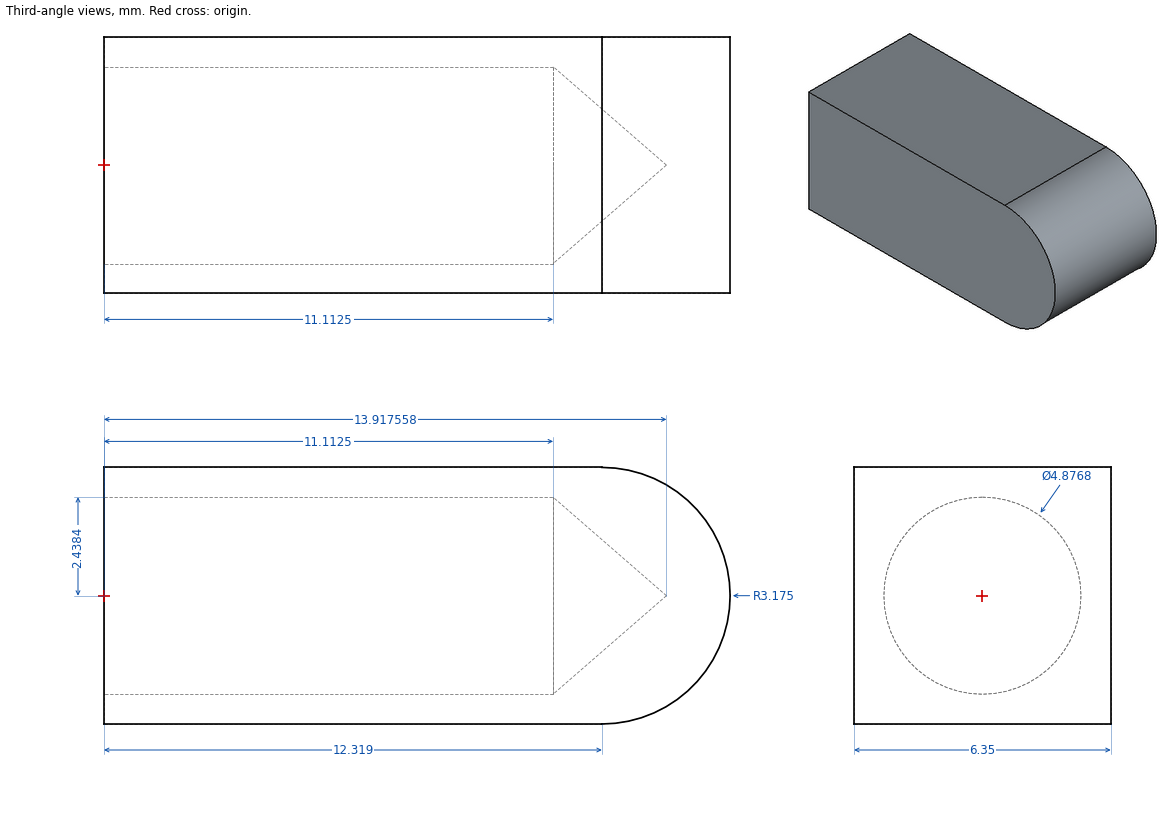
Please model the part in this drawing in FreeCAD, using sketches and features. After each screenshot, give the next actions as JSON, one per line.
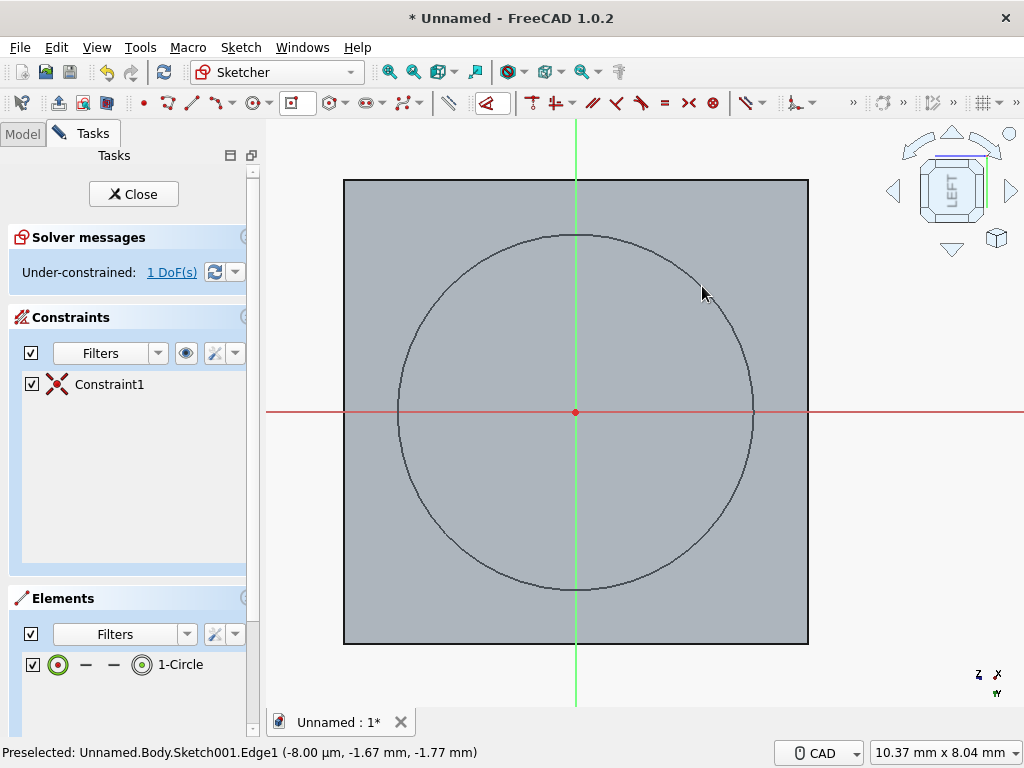
{"action": "key", "text": "d"}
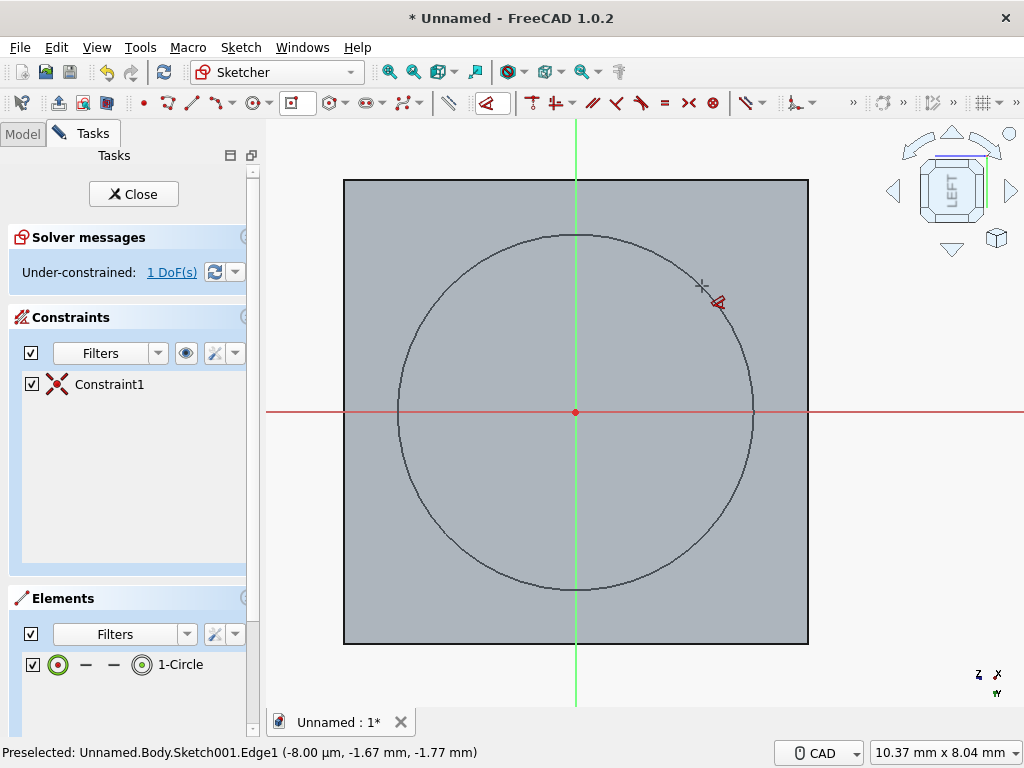
{"action": "left_click", "coordinate": [701, 286]}
{"action": "left_click", "coordinate": [724, 263]}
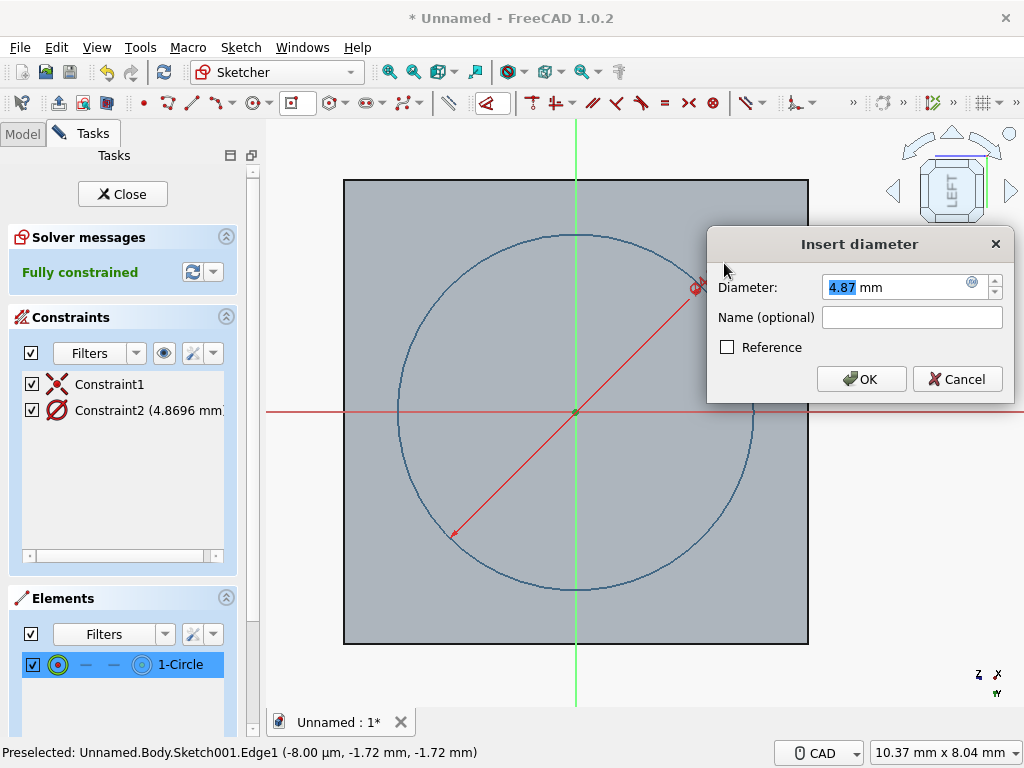
{"action": "type", "text": "4.8768"}
{"action": "key", "text": "Return"}
{"action": "key", "text": "Escape"}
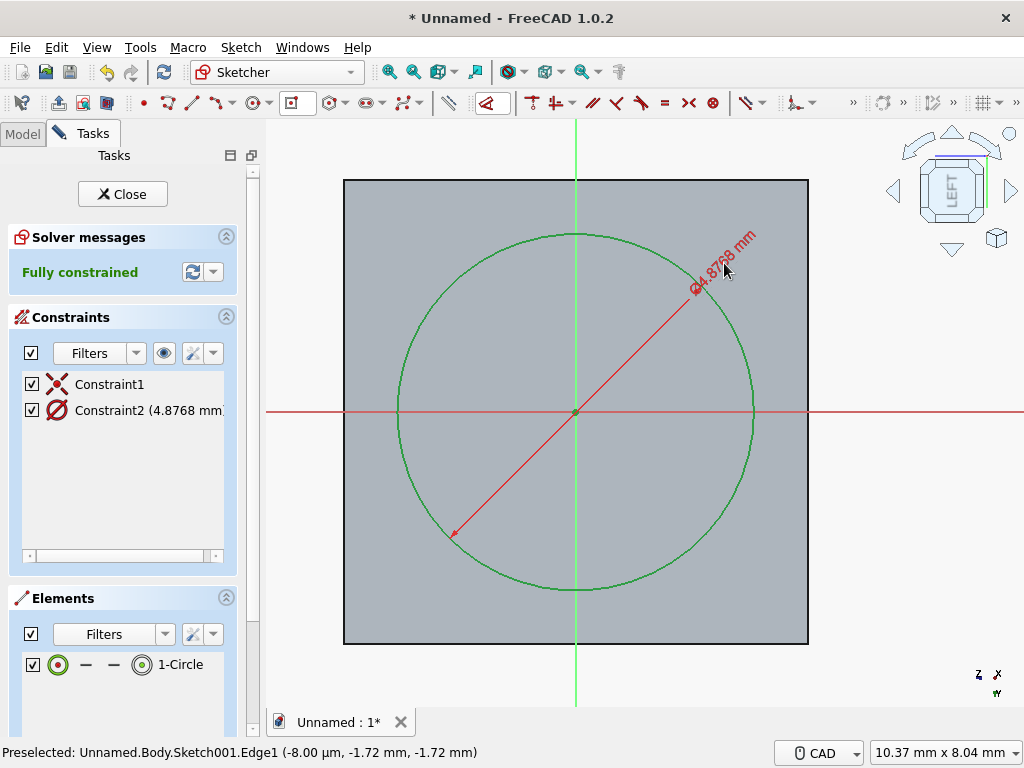
{"action": "left_click", "coordinate": [123, 194]}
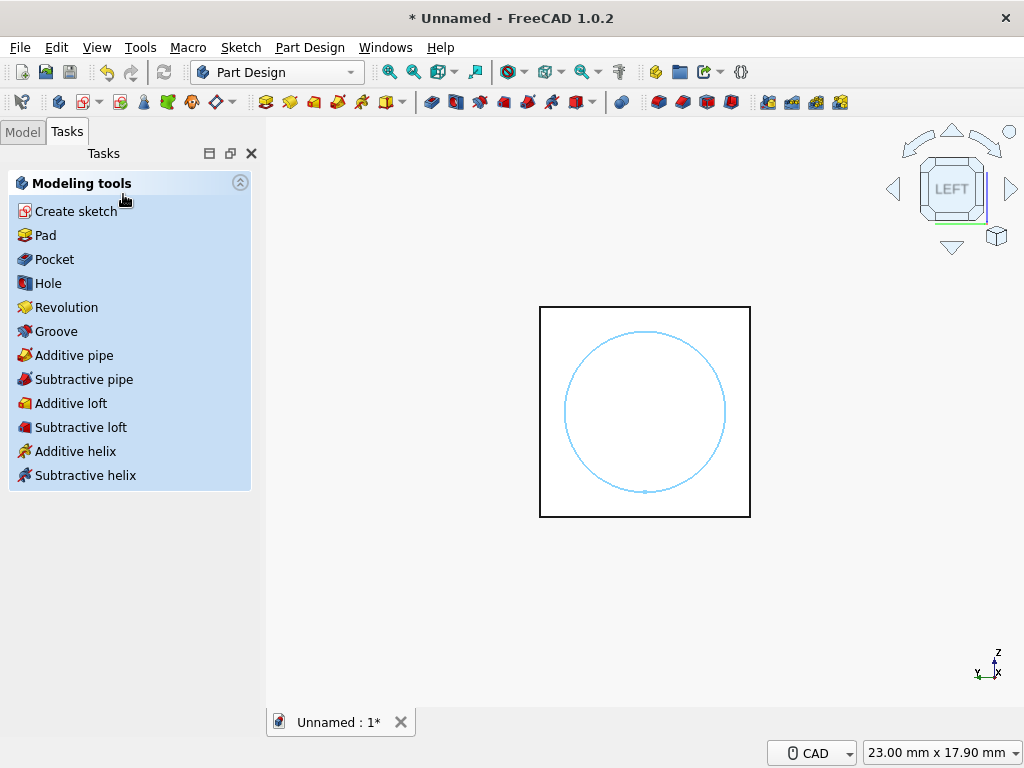
{"action": "left_click", "coordinate": [432, 102]}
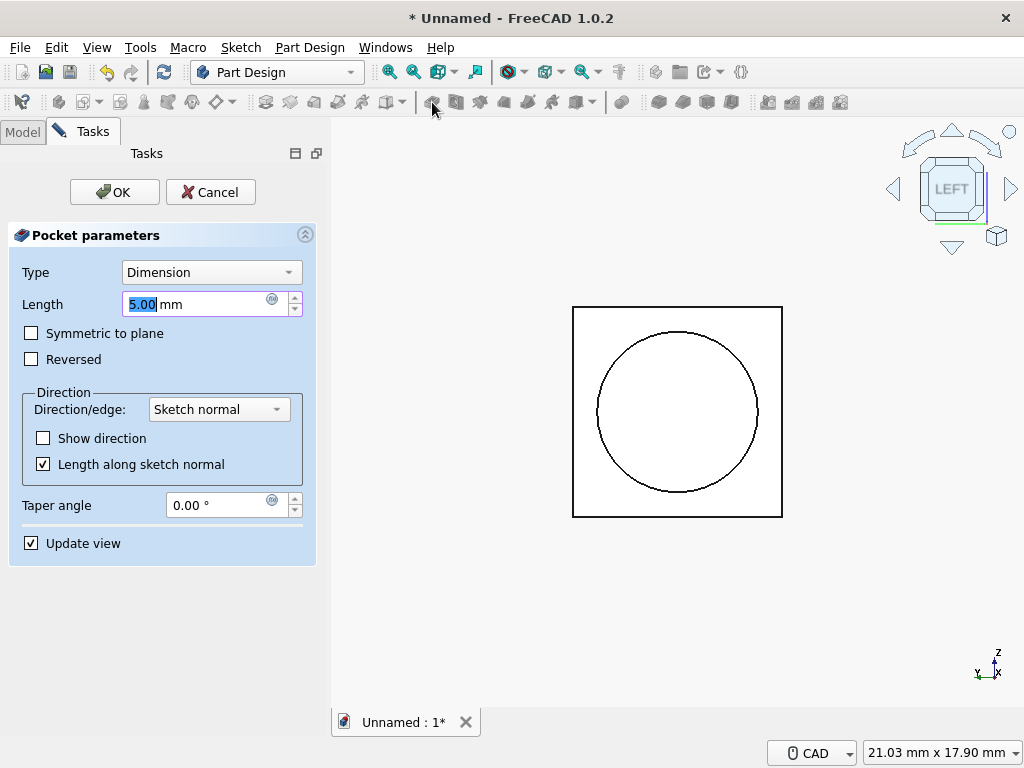
{"action": "type", "text": "11.1125"}
{"action": "key", "text": "Tab"}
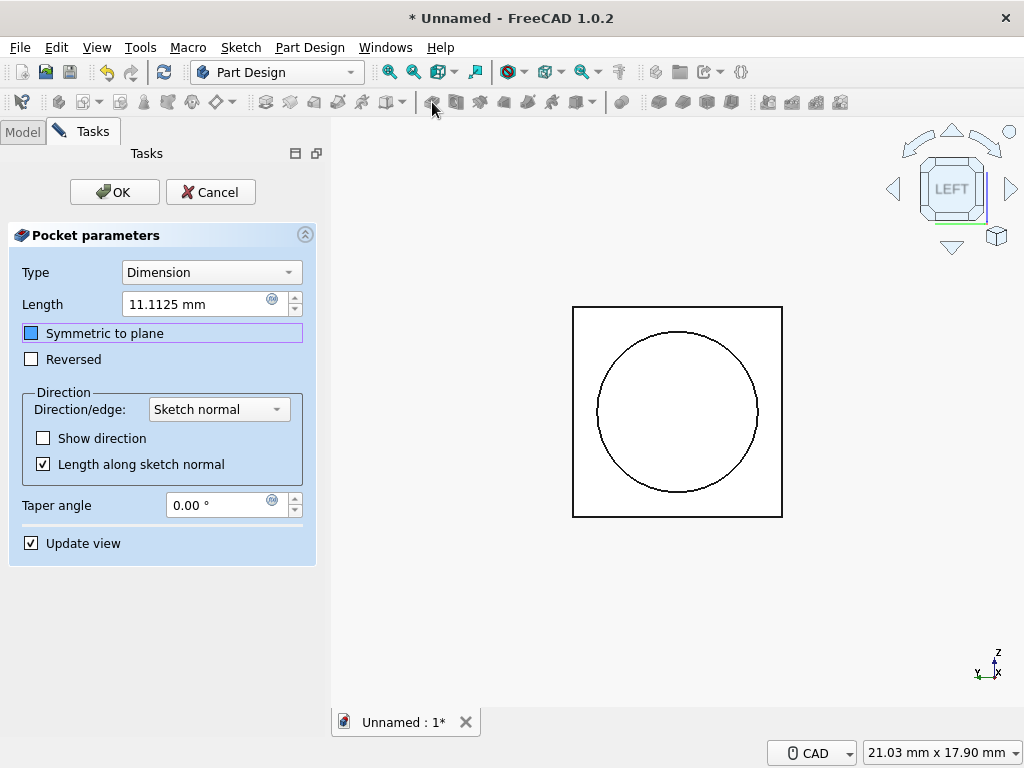
{"action": "left_click", "coordinate": [115, 192]}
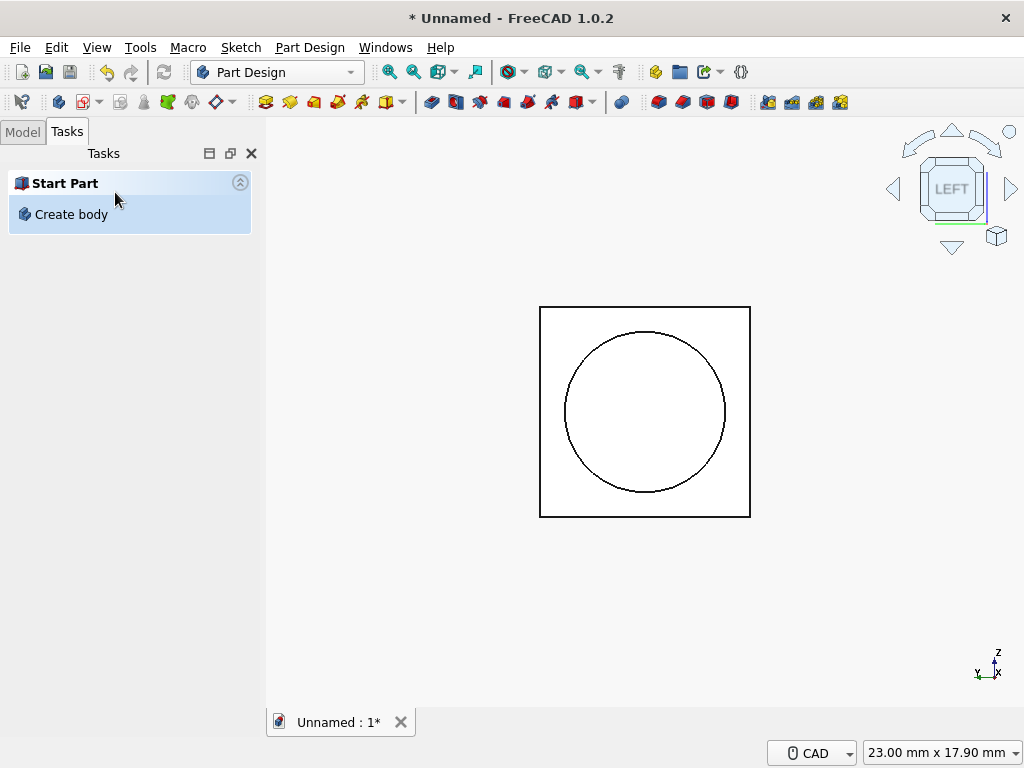
{"action": "key", "text": "v f"}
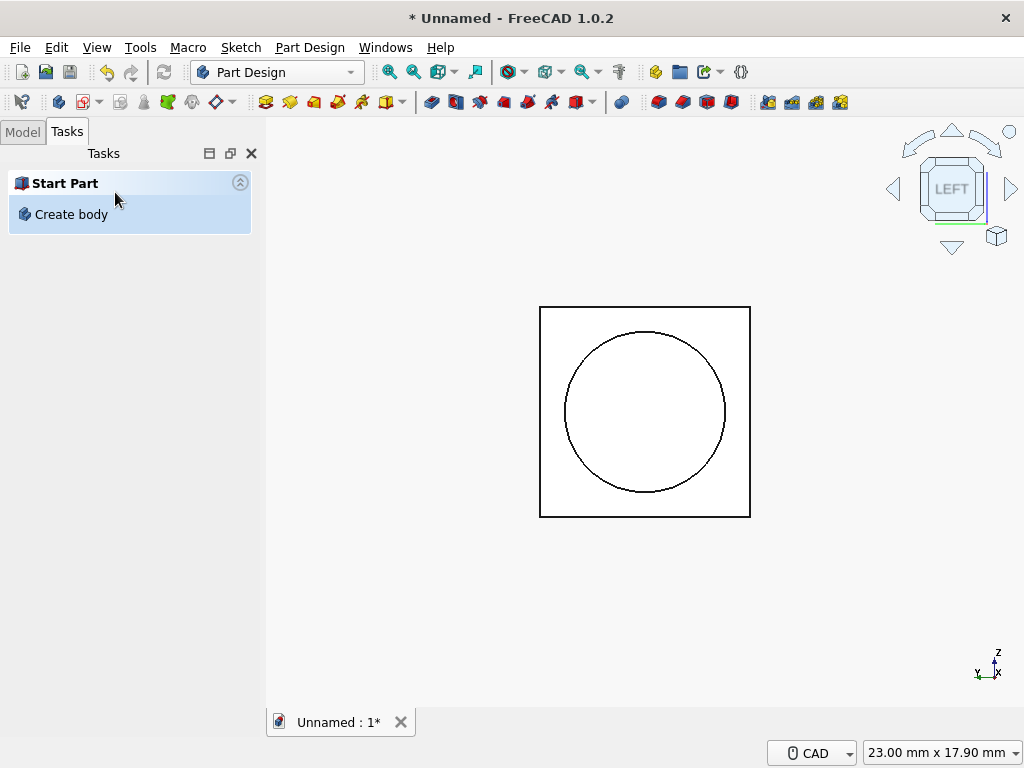
{"action": "left_click", "coordinate": [84, 102]}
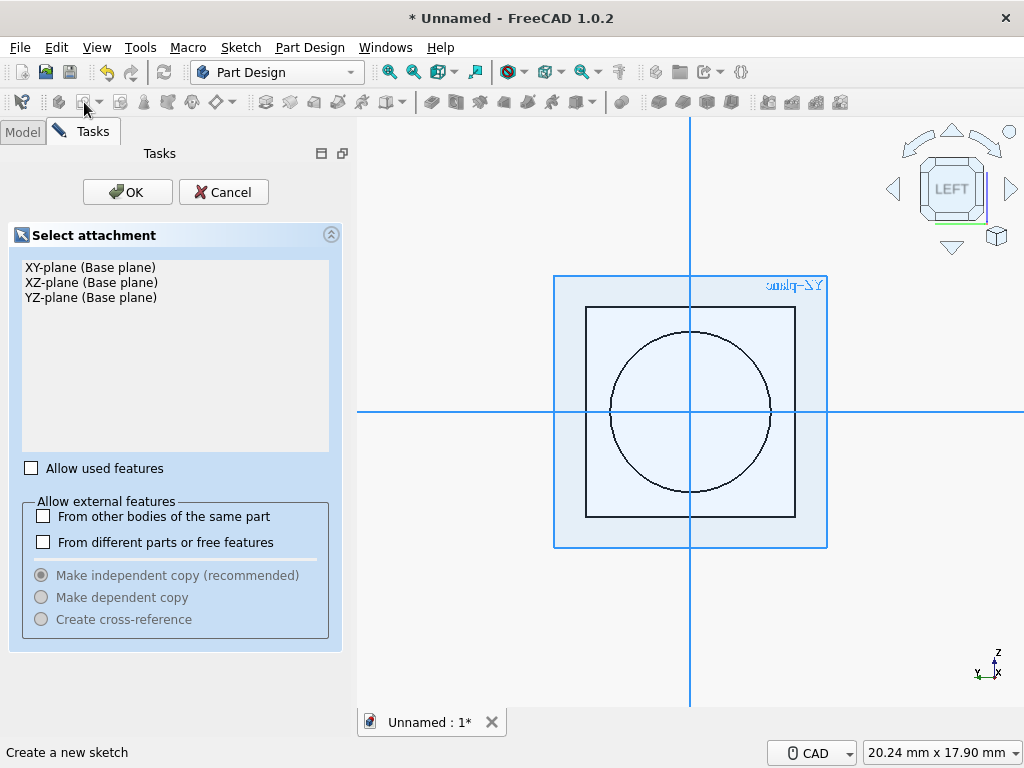
{"action": "left_click", "coordinate": [82, 282]}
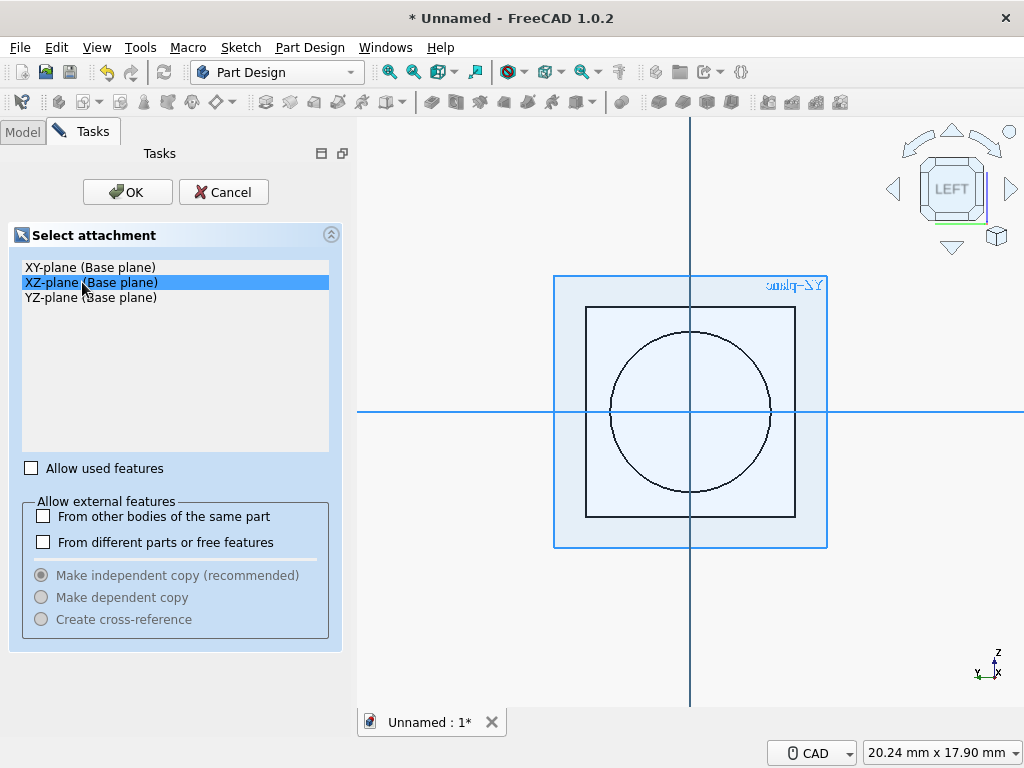
{"action": "left_click", "coordinate": [128, 192]}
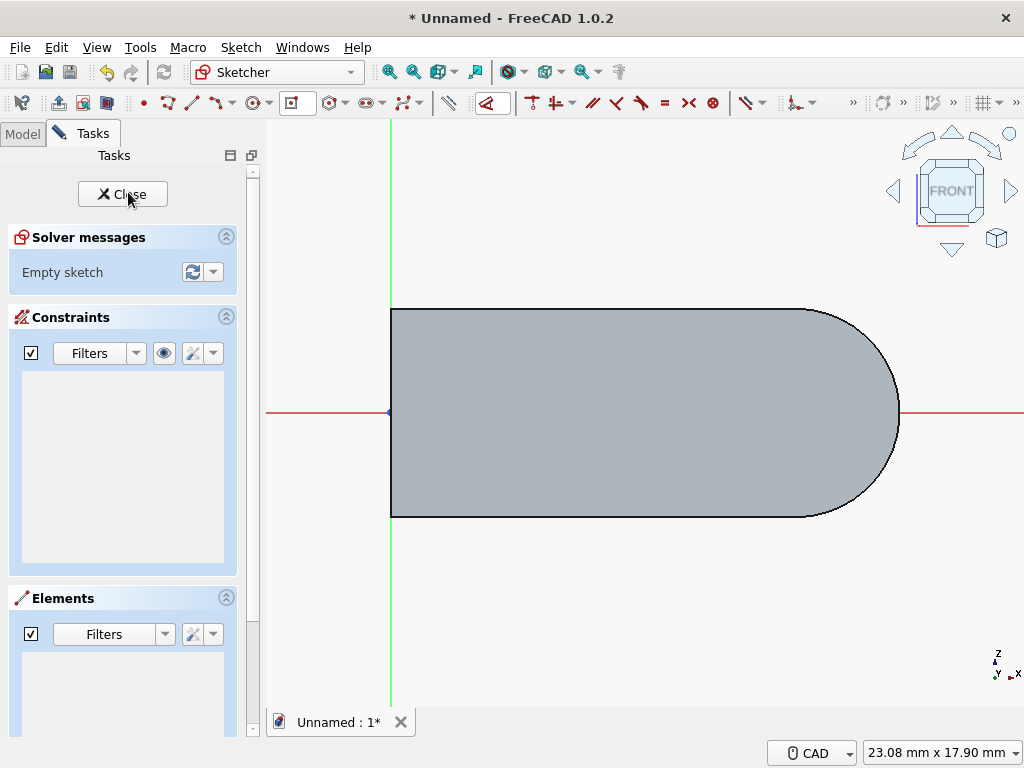
{"action": "left_click", "coordinate": [108, 104]}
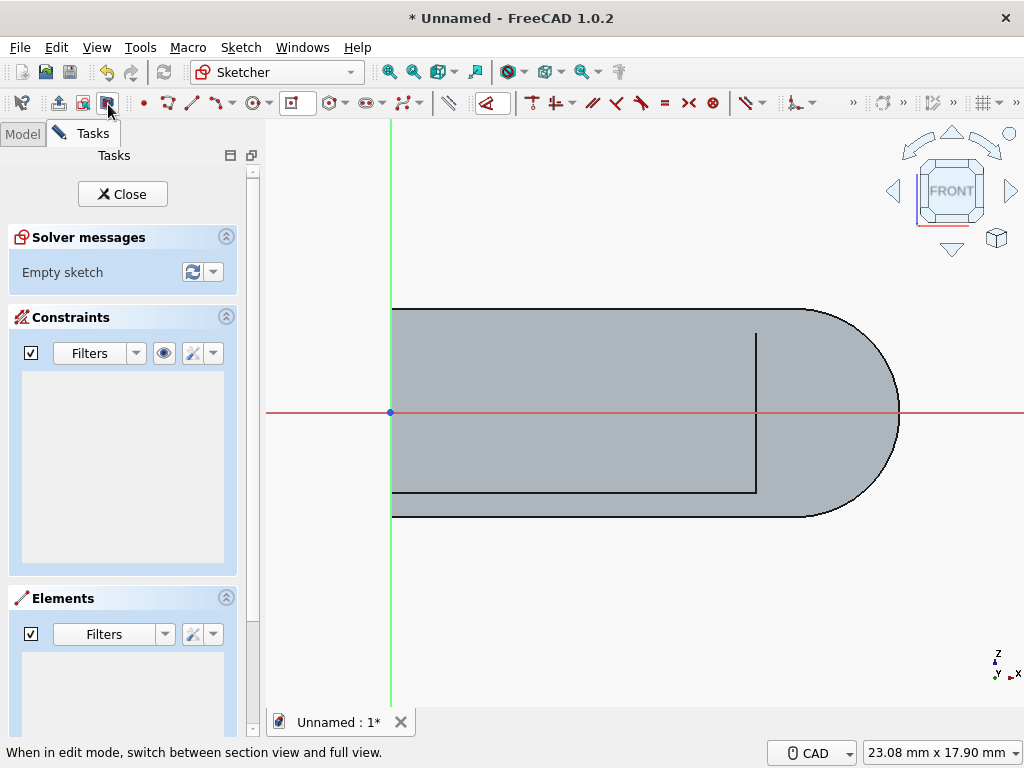
{"action": "scroll", "coordinate": [383, 594], "scroll_direction": "down", "scroll_amount": 1}